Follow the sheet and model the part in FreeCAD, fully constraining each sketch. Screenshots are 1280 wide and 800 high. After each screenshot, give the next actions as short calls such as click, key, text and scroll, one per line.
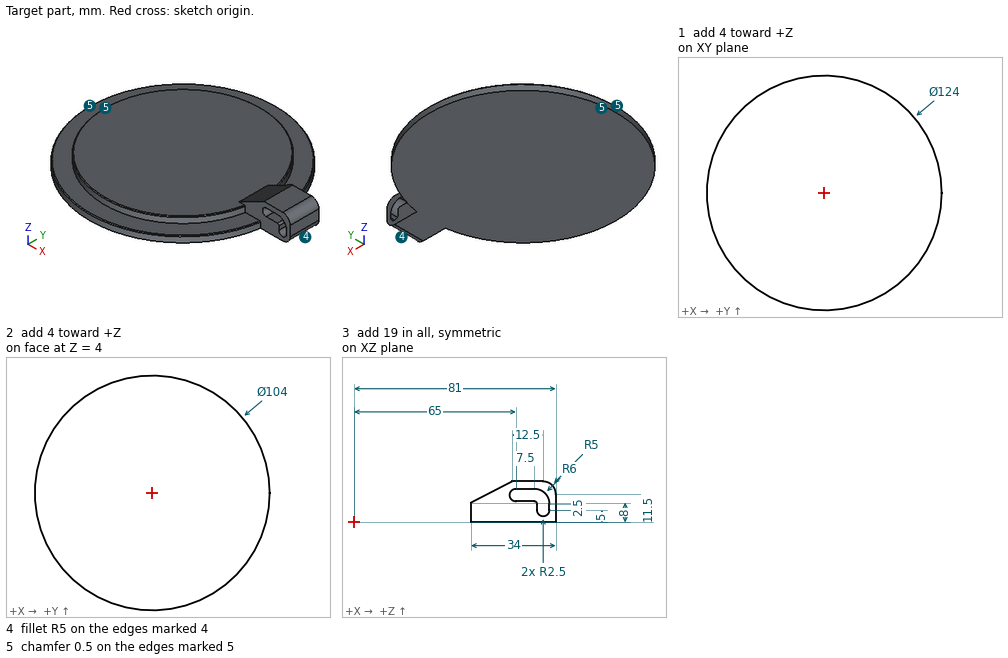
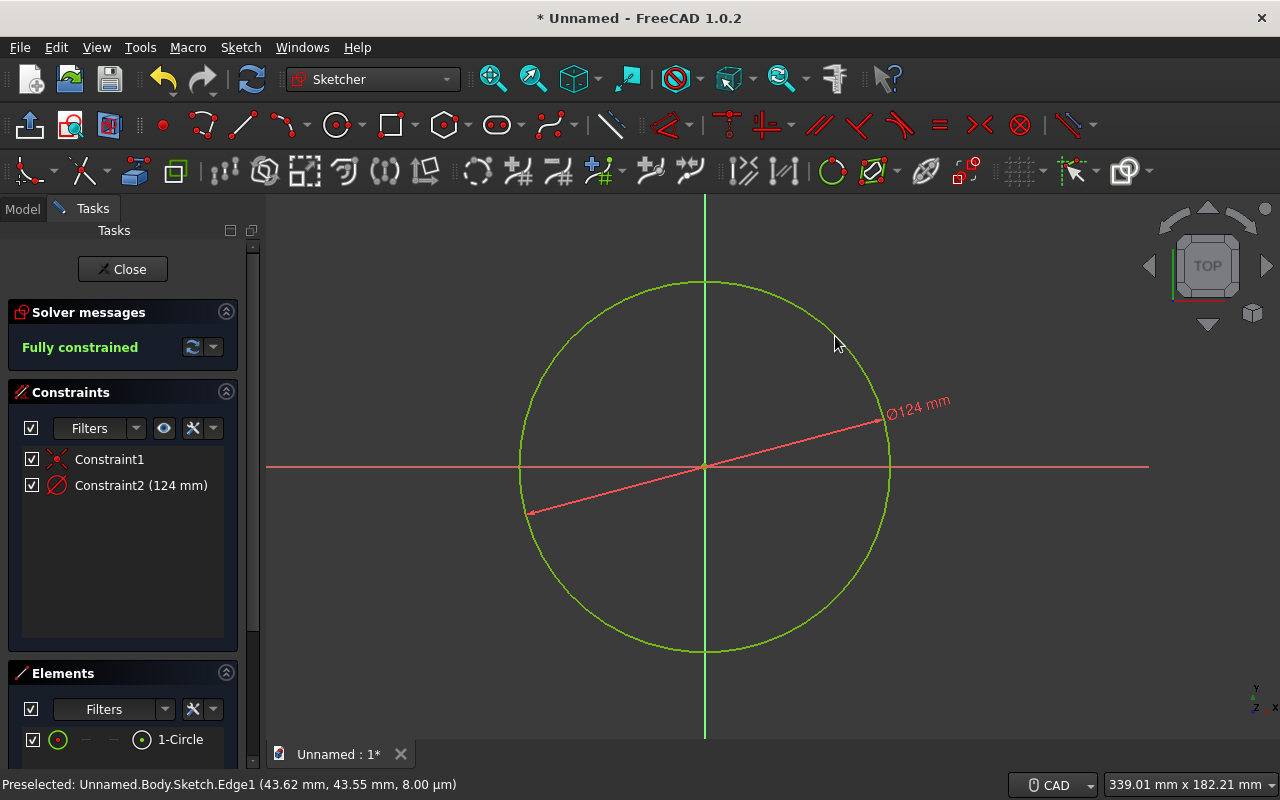
click(123, 269)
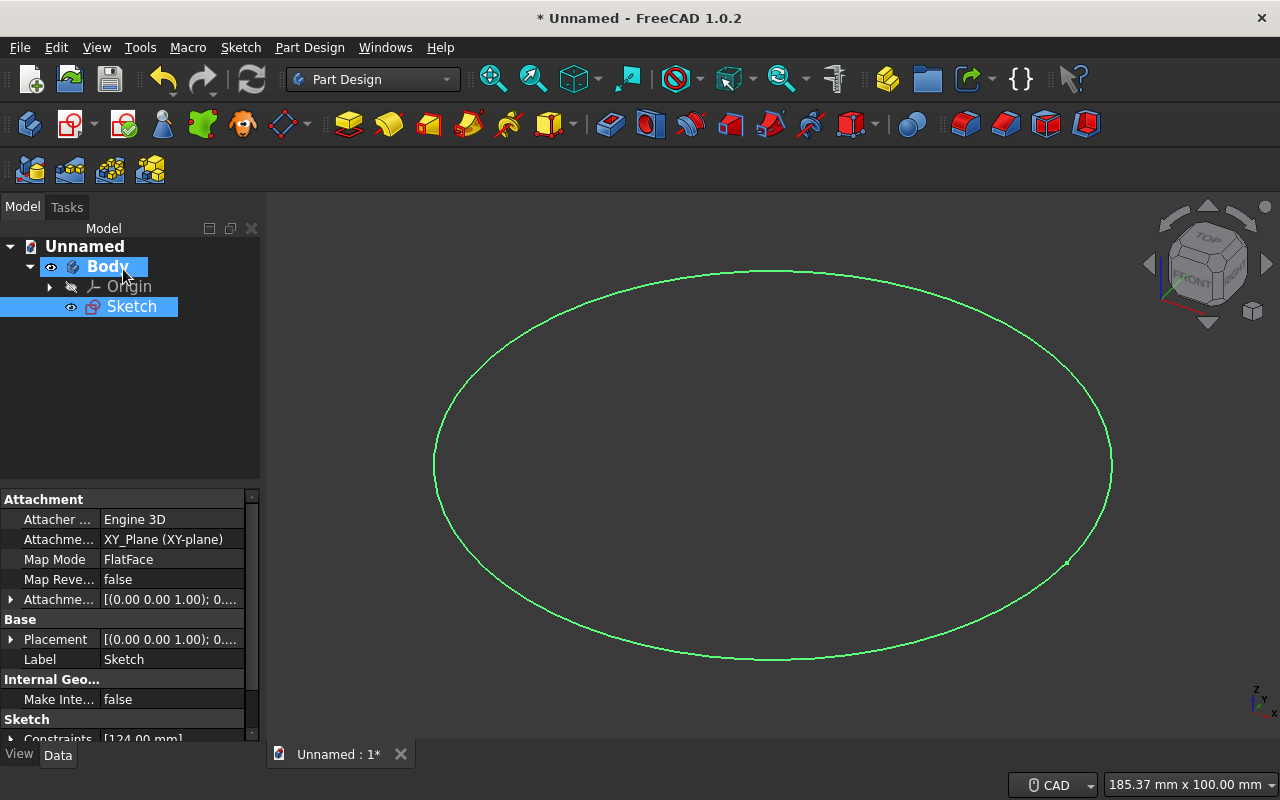
click(350, 124)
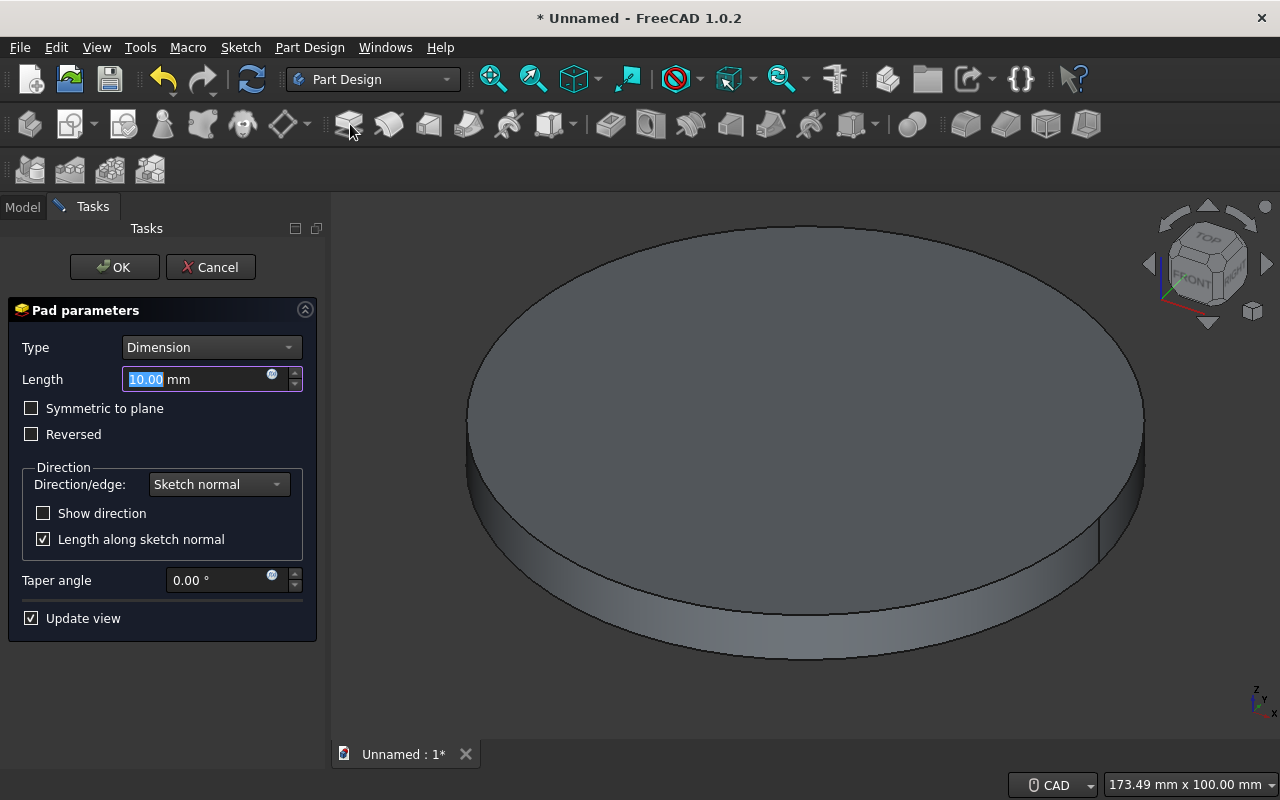
text(4)
key(Tab)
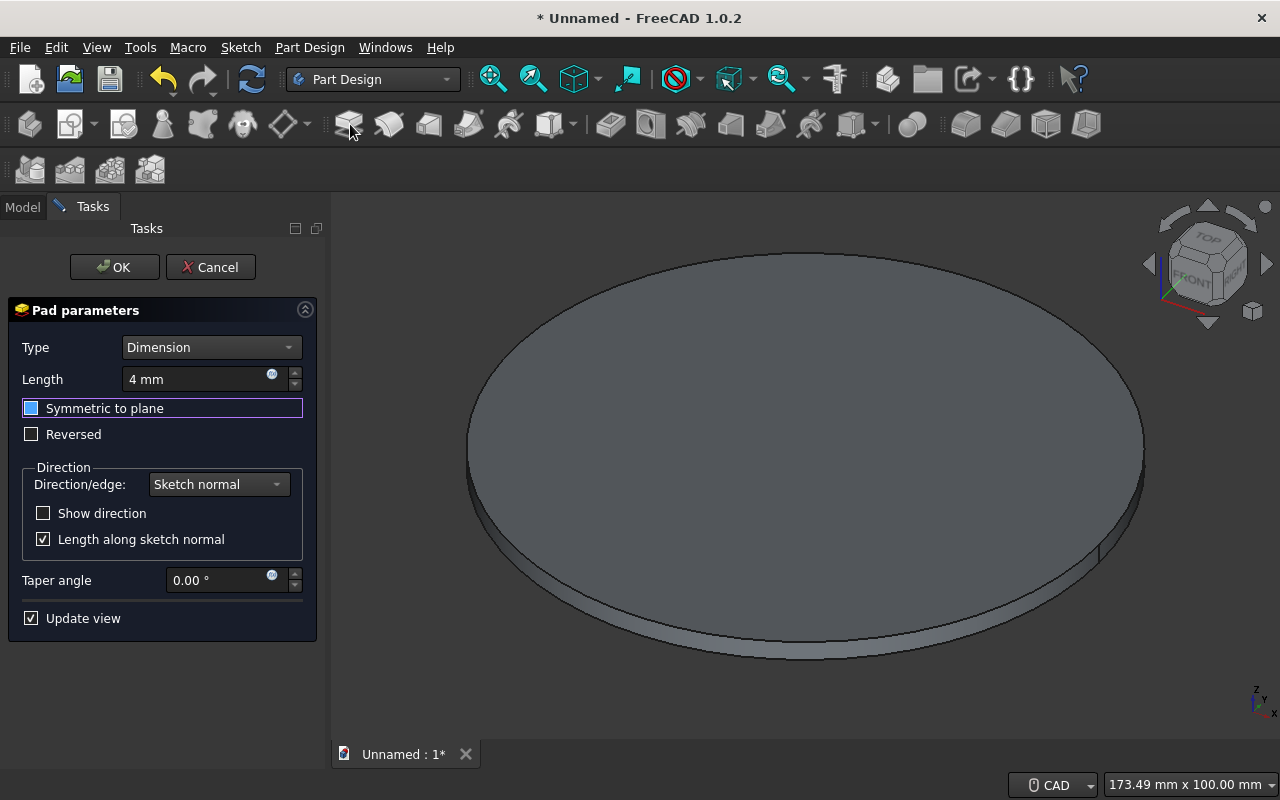
click(115, 267)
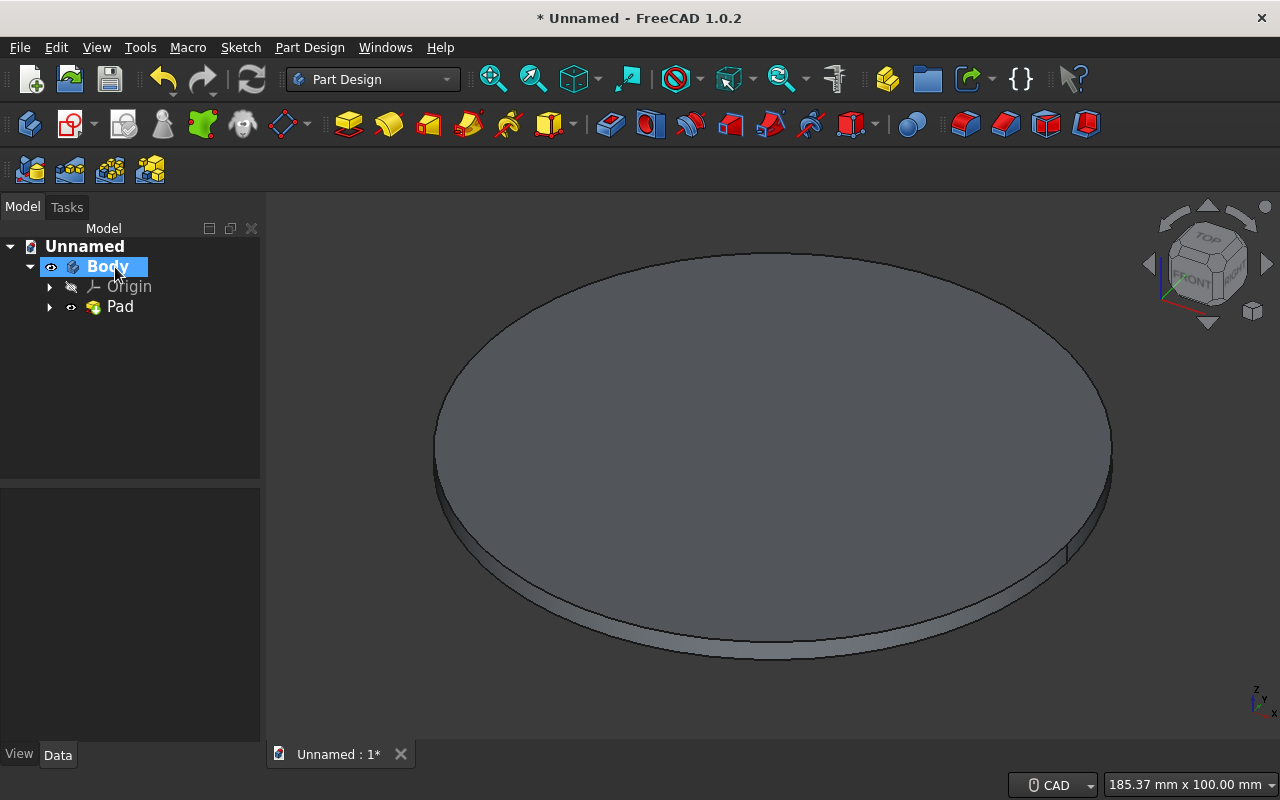
key(v)
key(f)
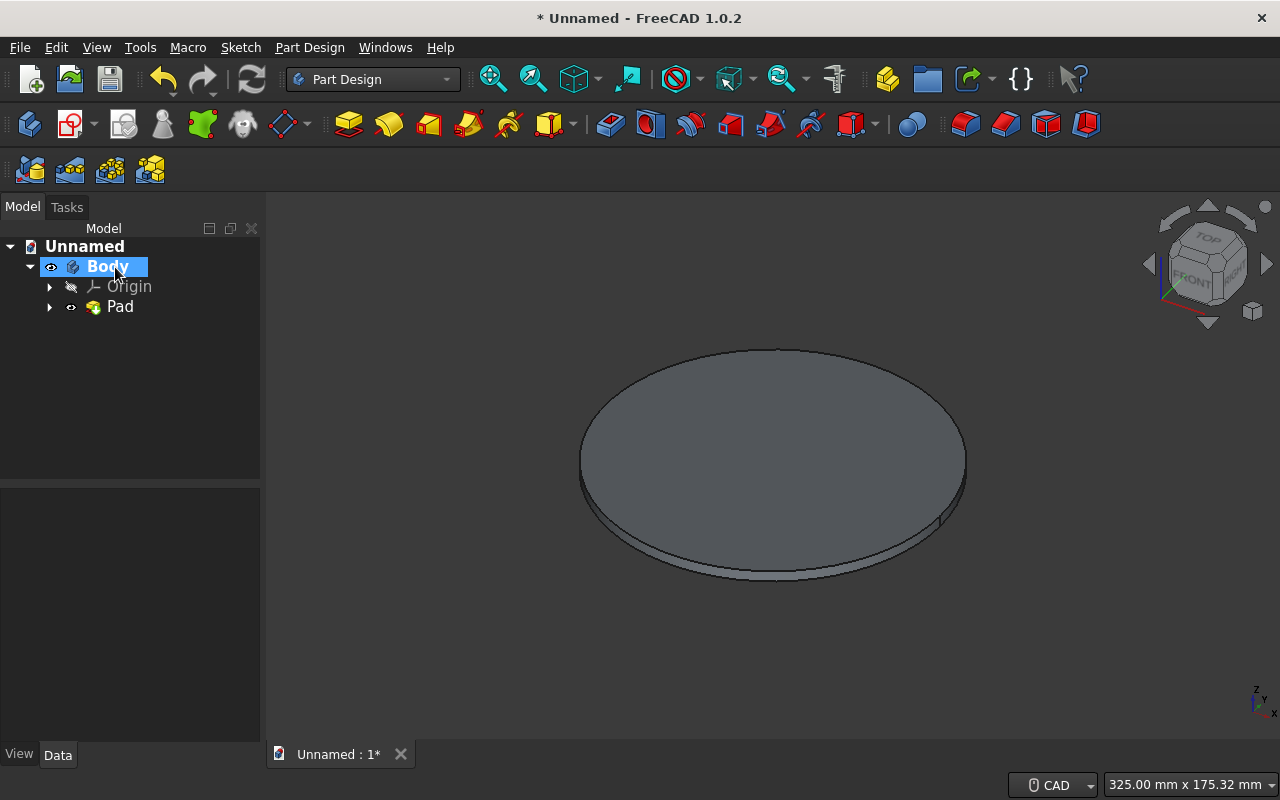
click(773, 459)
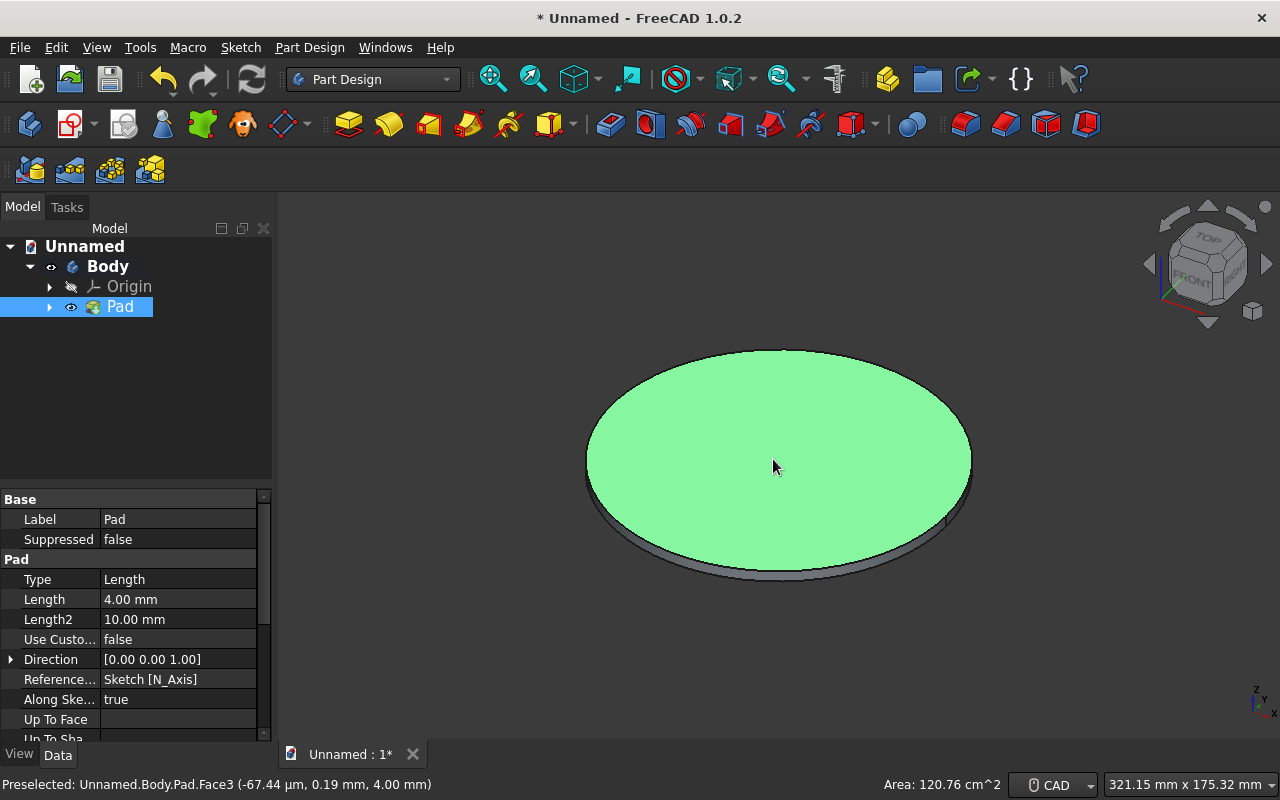
click(70, 124)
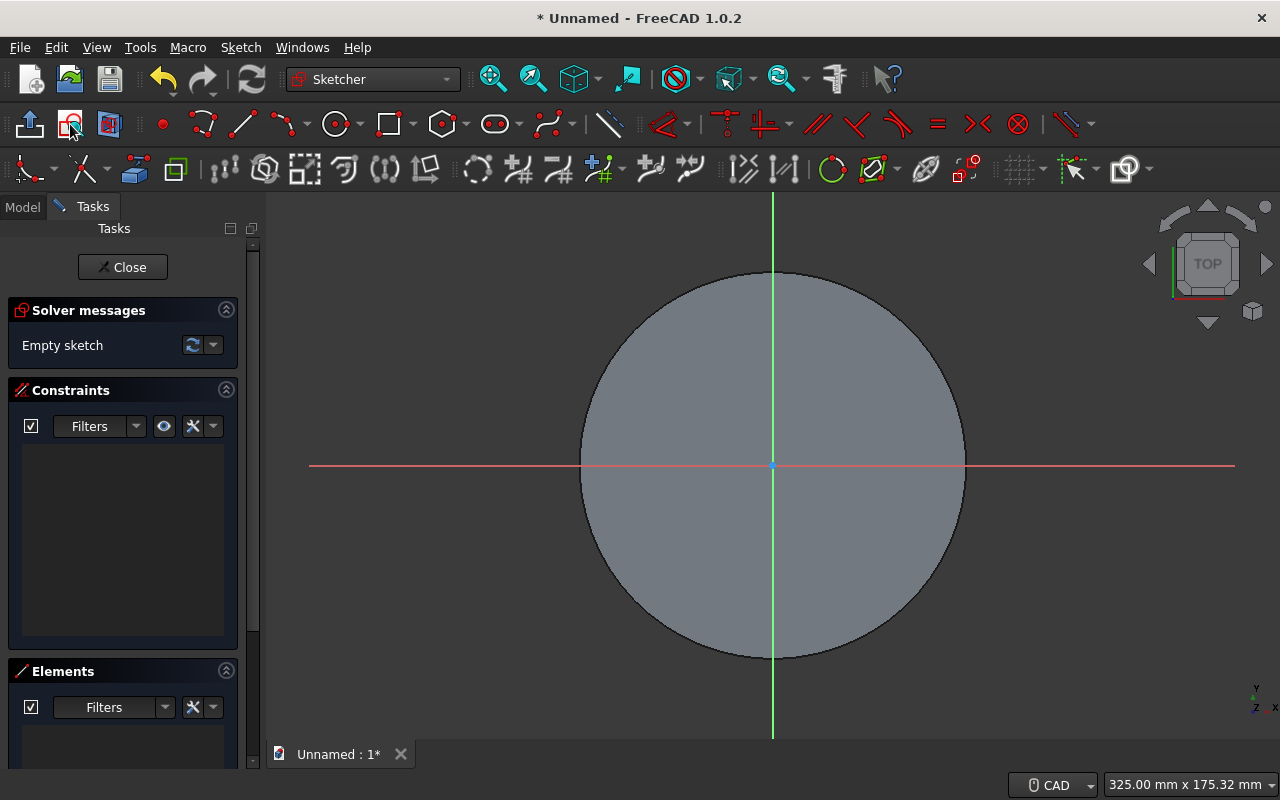
click(336, 124)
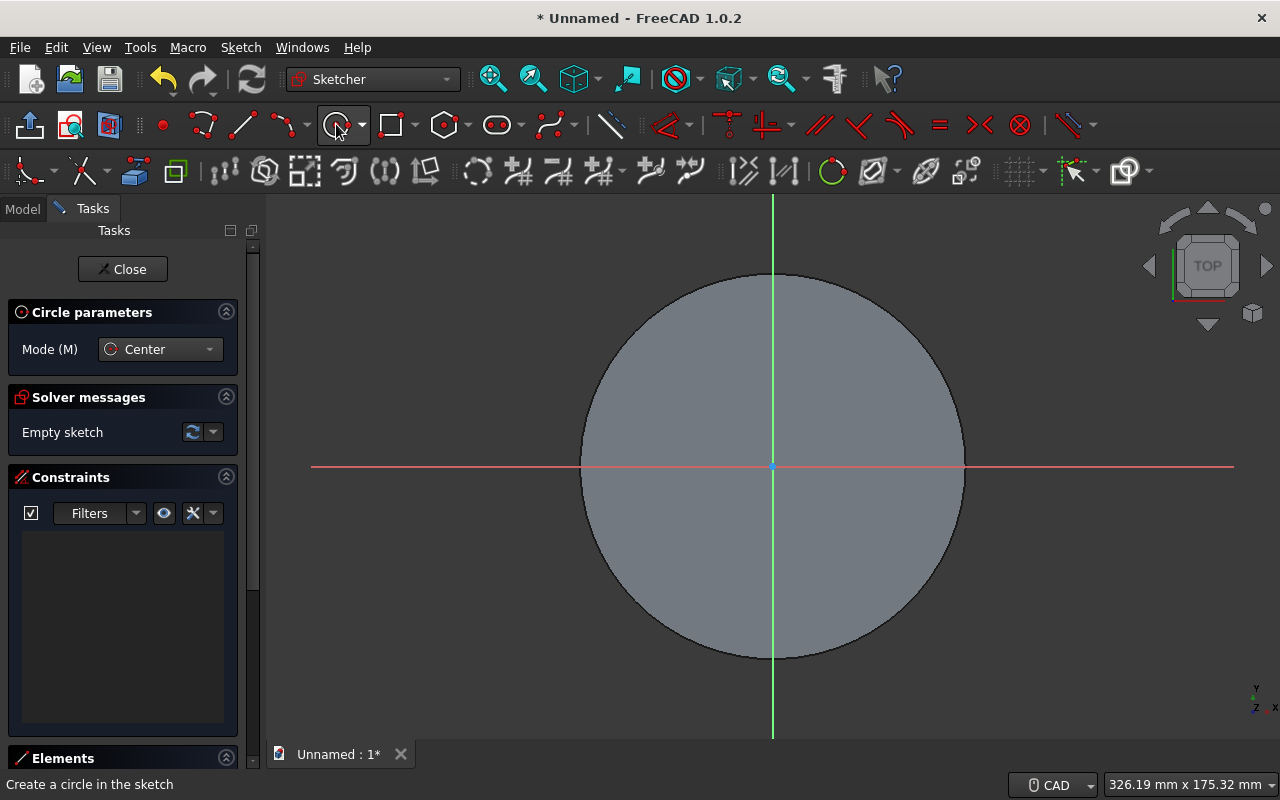
click(773, 466)
click(887, 352)
key(Escape)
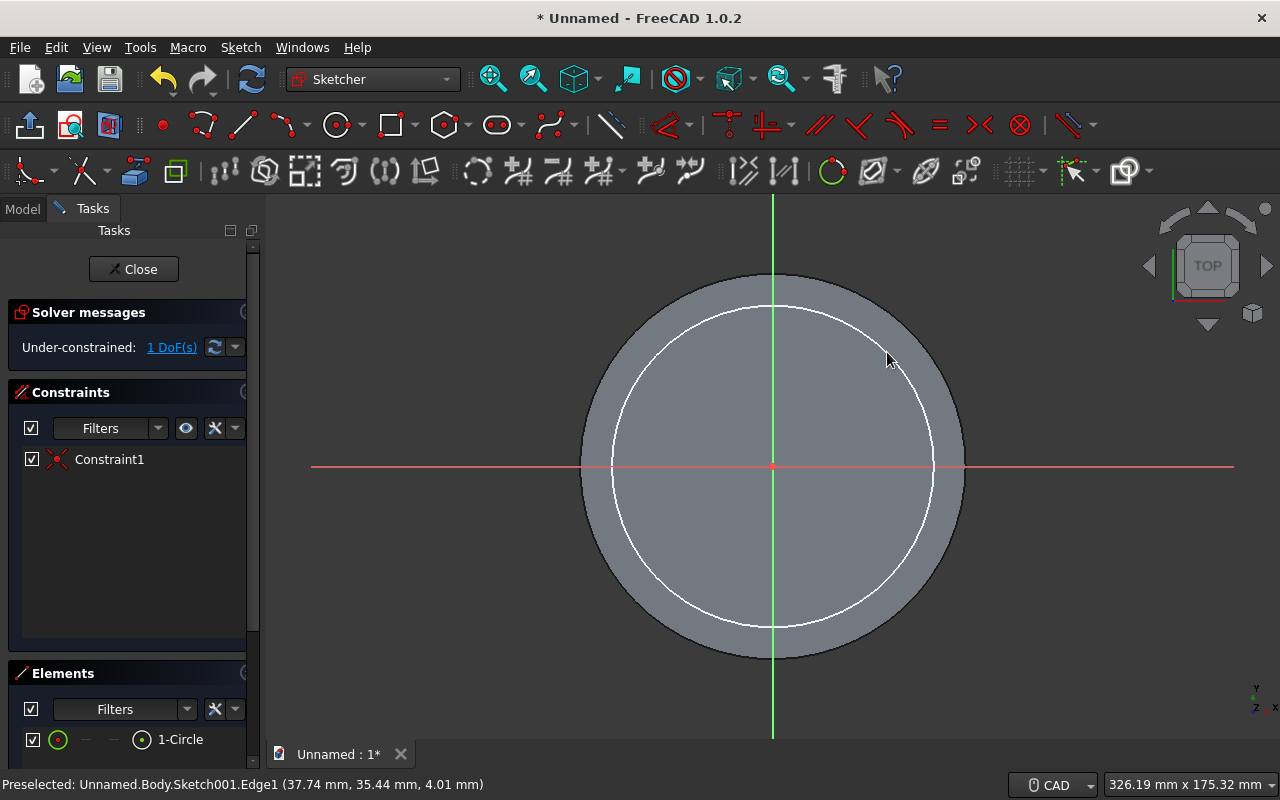
click(886, 352)